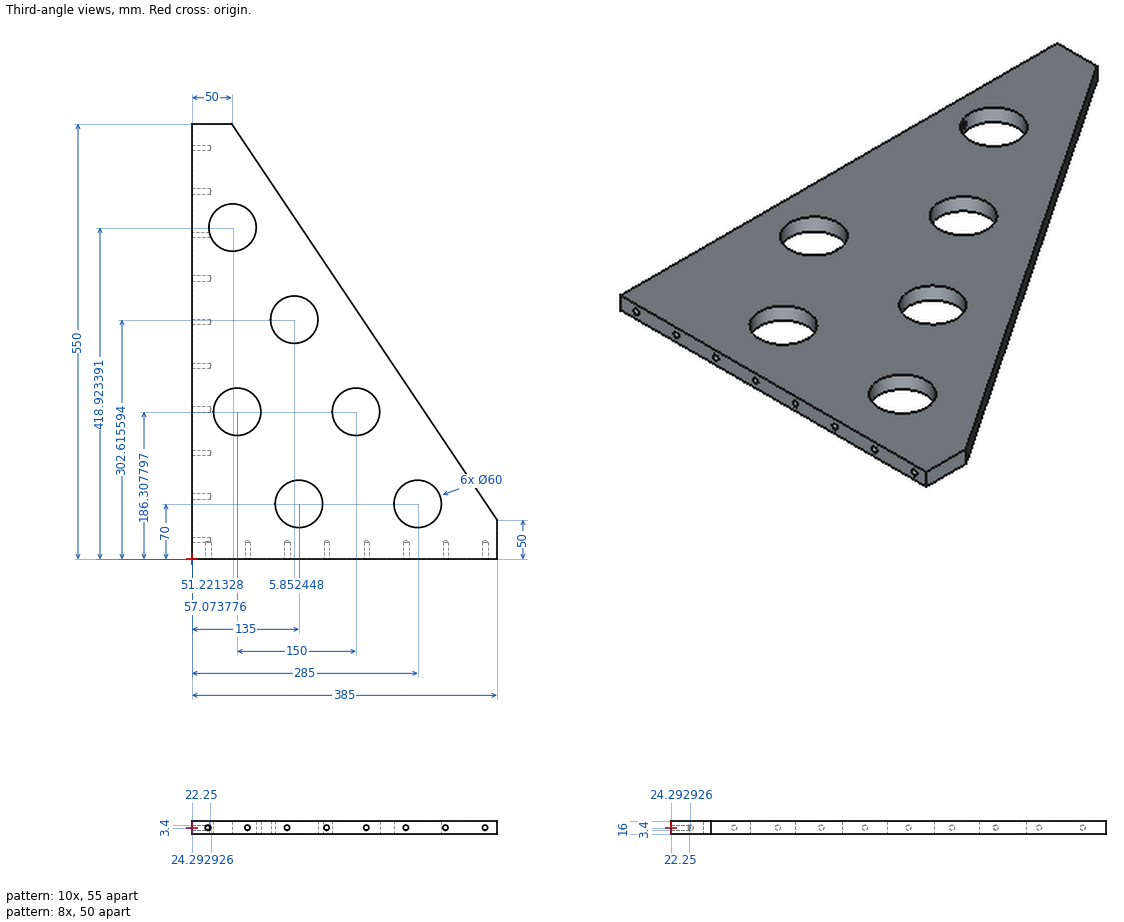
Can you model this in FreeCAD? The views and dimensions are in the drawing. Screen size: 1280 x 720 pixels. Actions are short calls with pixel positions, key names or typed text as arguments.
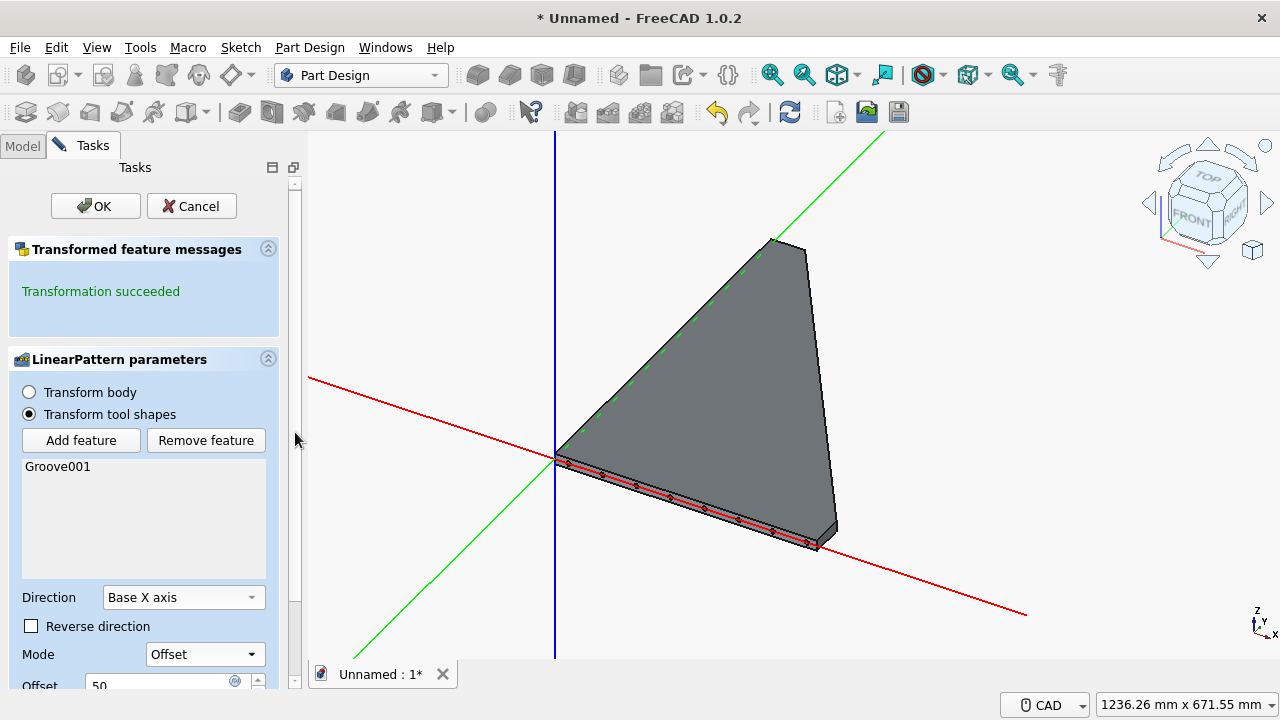
click(96, 206)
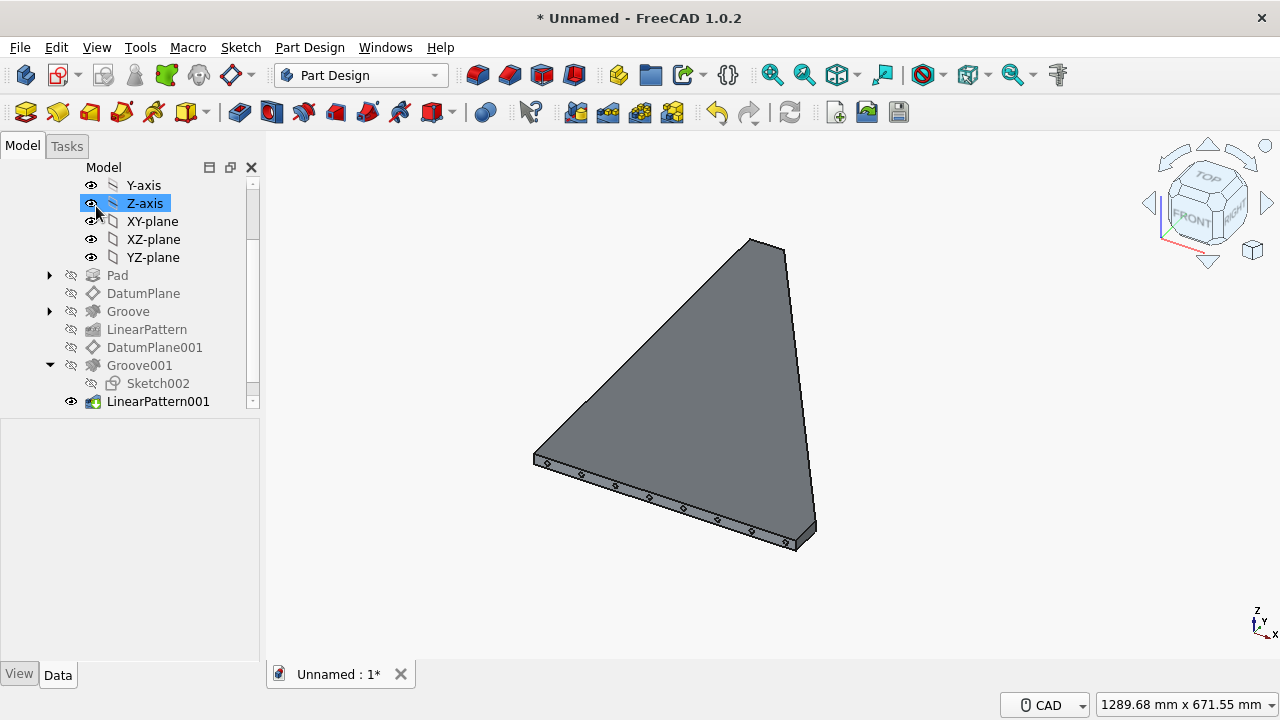
key(5)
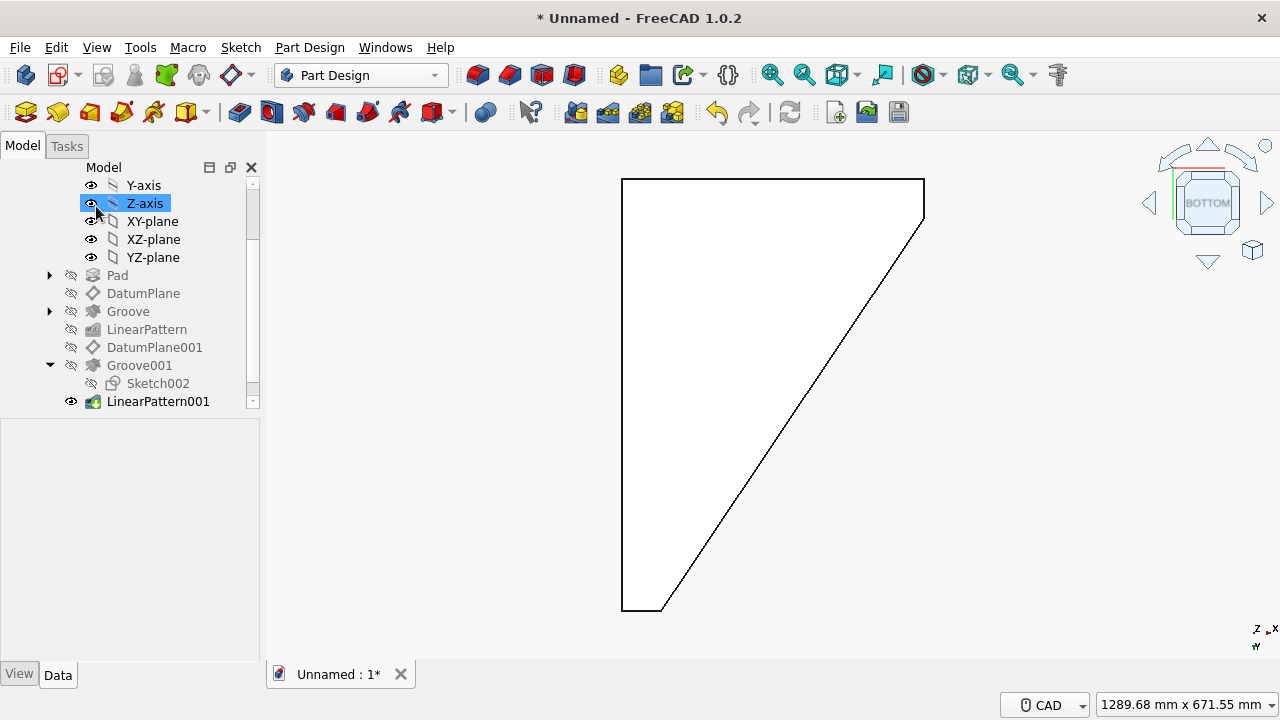
click(730, 332)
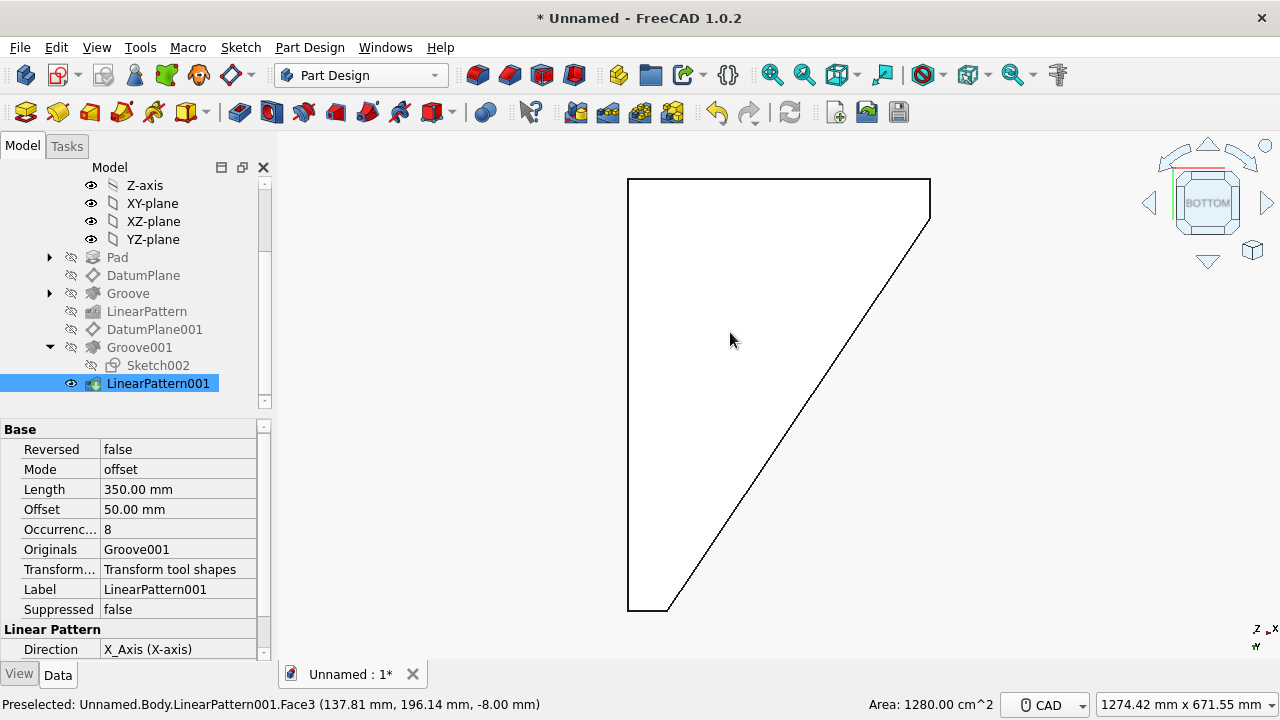
click(58, 76)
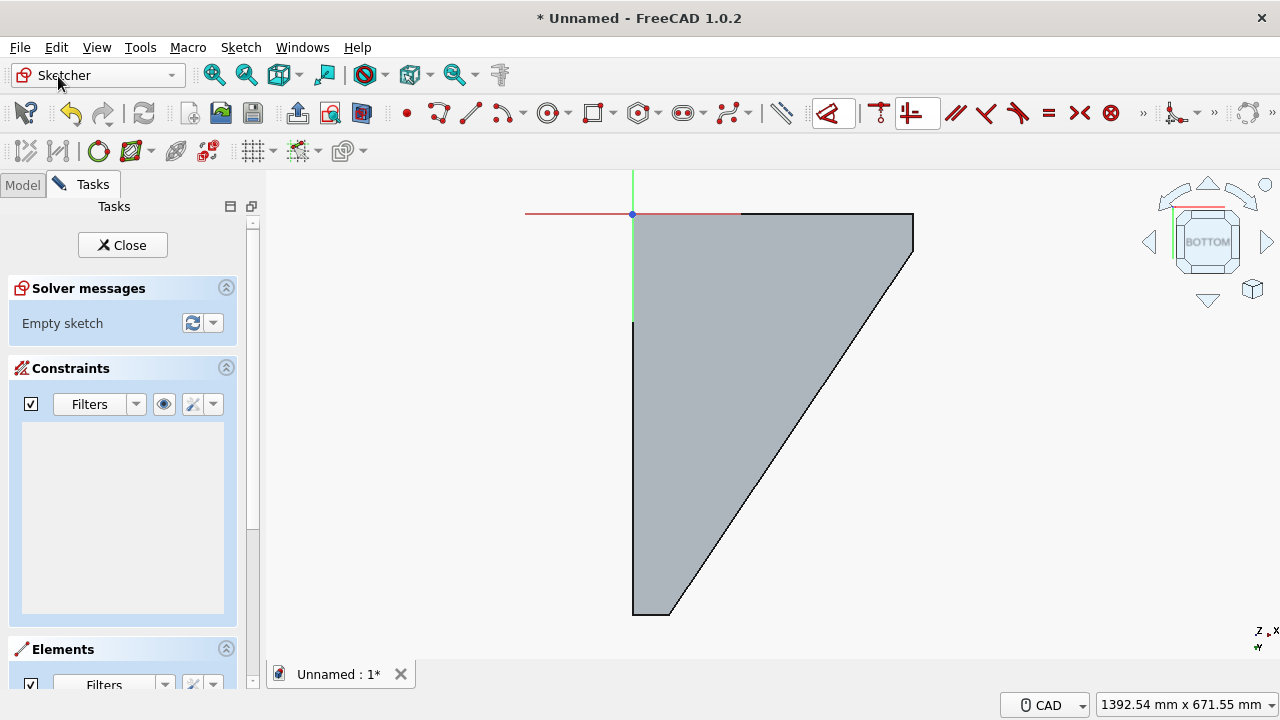
scroll(510, 581, down, 1)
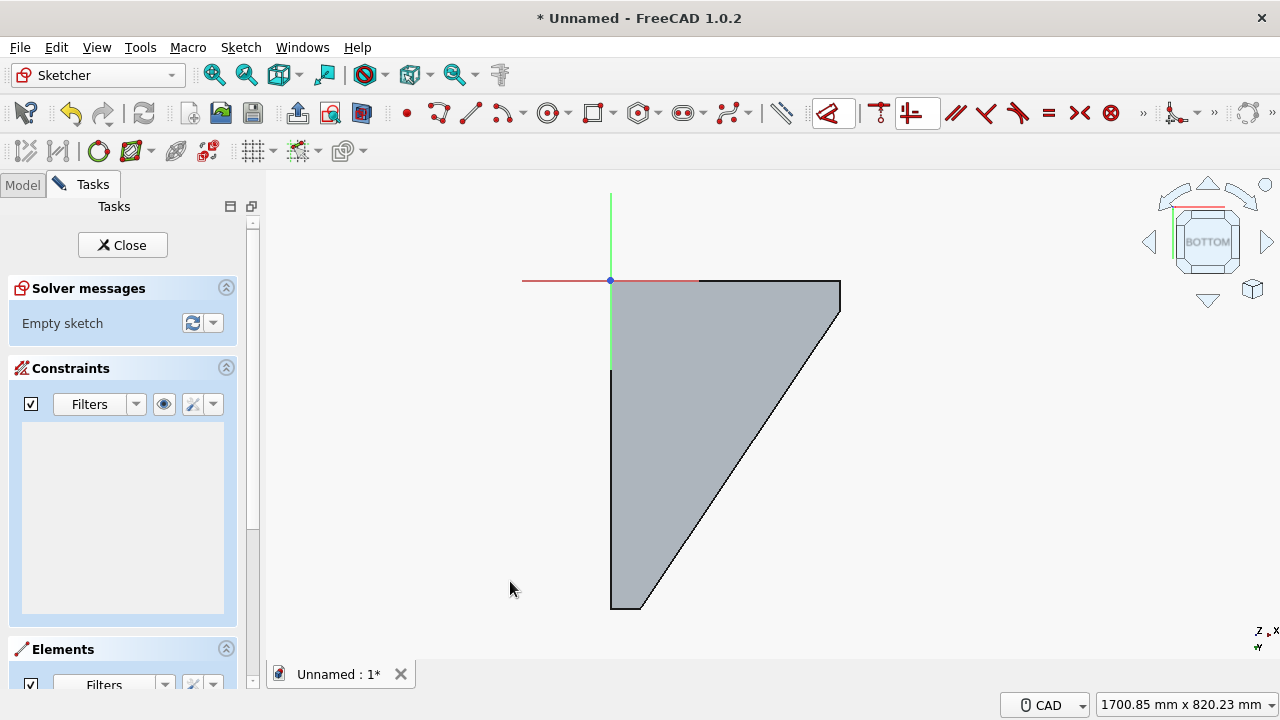
click(548, 114)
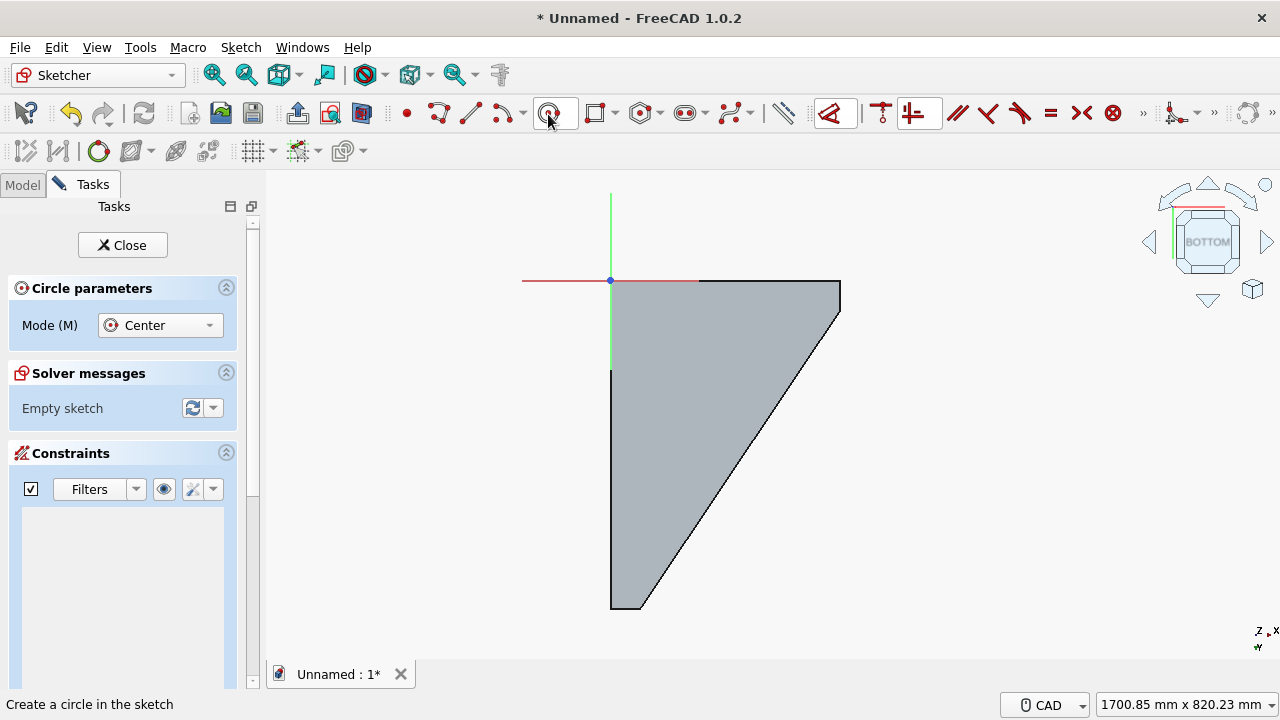
scroll(781, 323, up, 2)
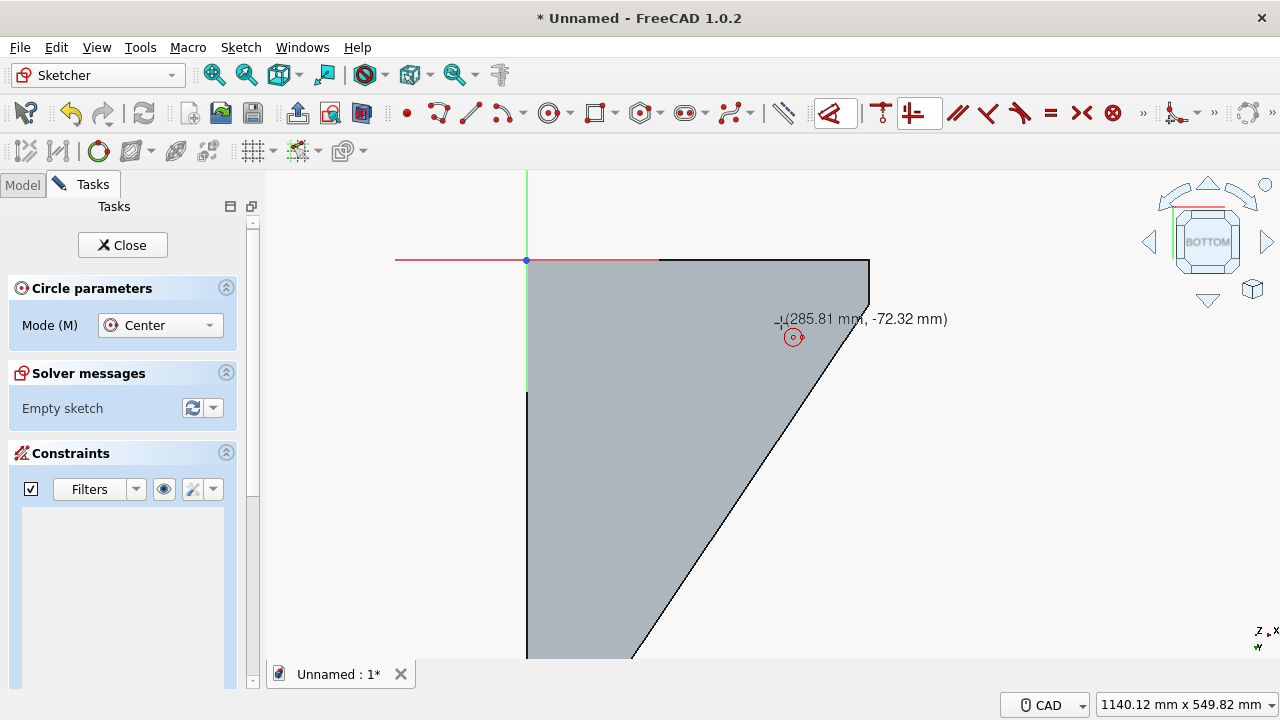
click(780, 322)
move(799, 303)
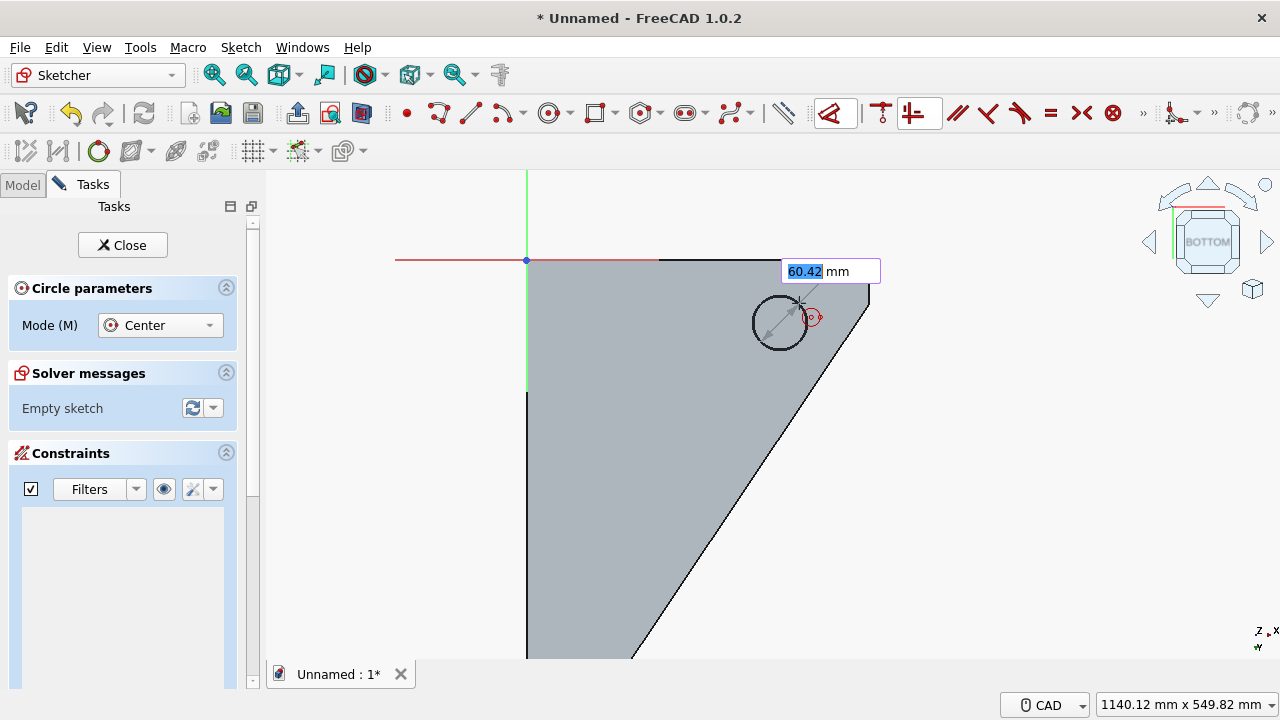
text(60)
key(Return)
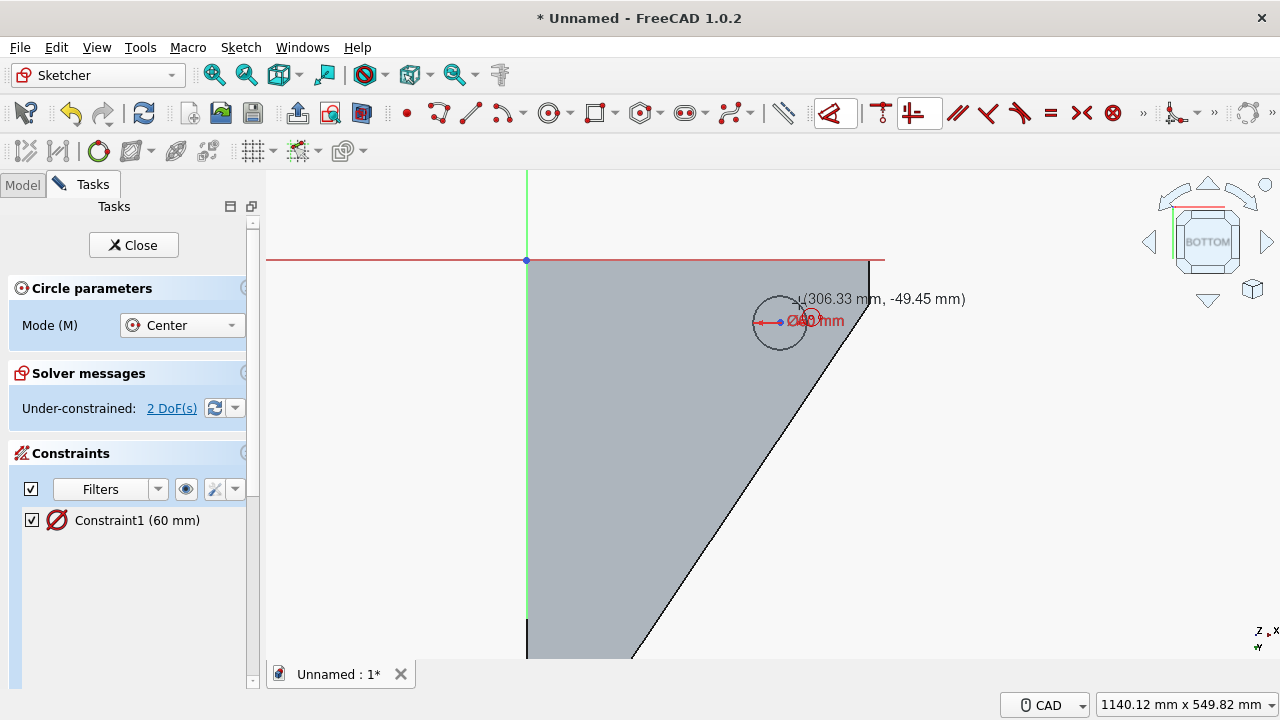
click(641, 529)
move(660, 510)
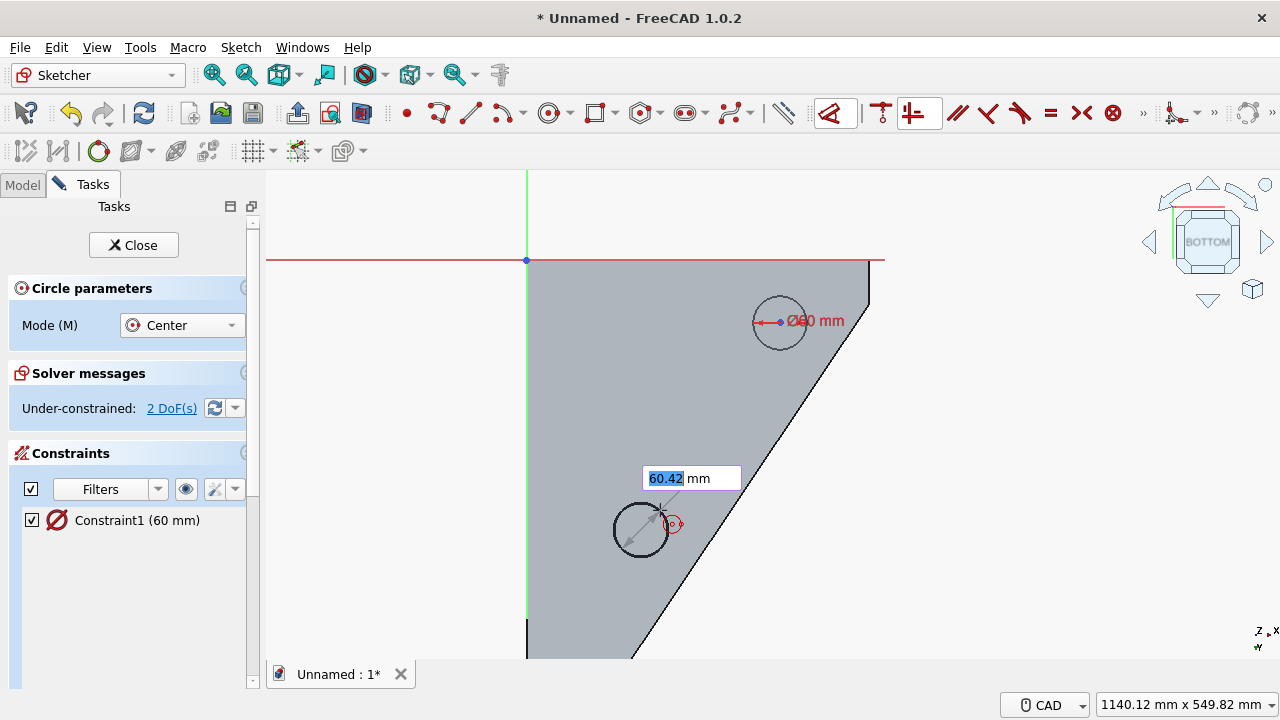
text(60)
key(Return)